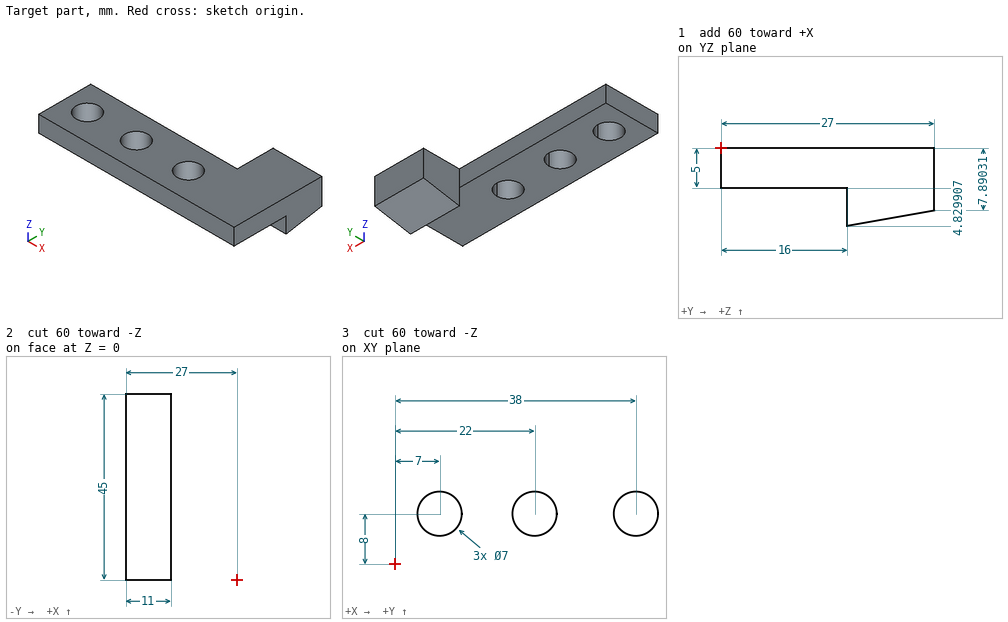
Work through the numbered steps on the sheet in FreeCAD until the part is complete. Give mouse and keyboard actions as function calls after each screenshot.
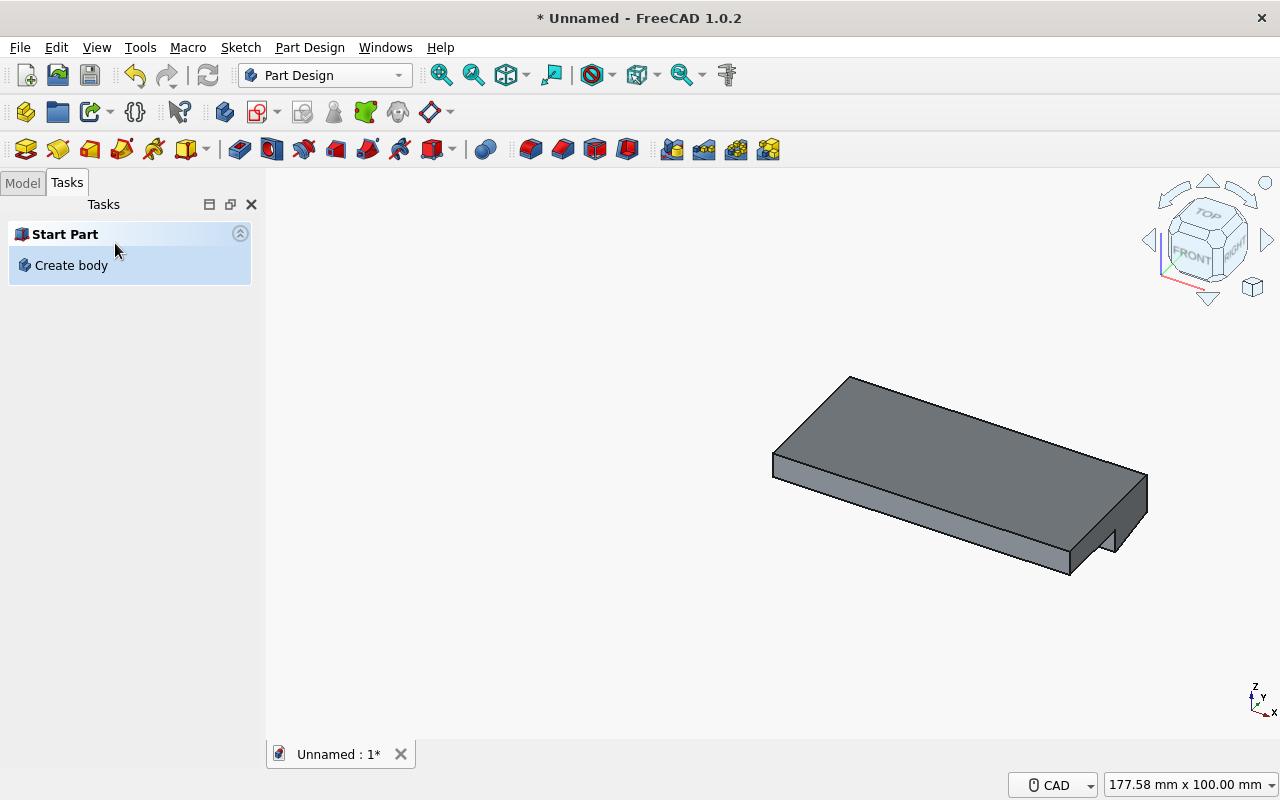
click(442, 76)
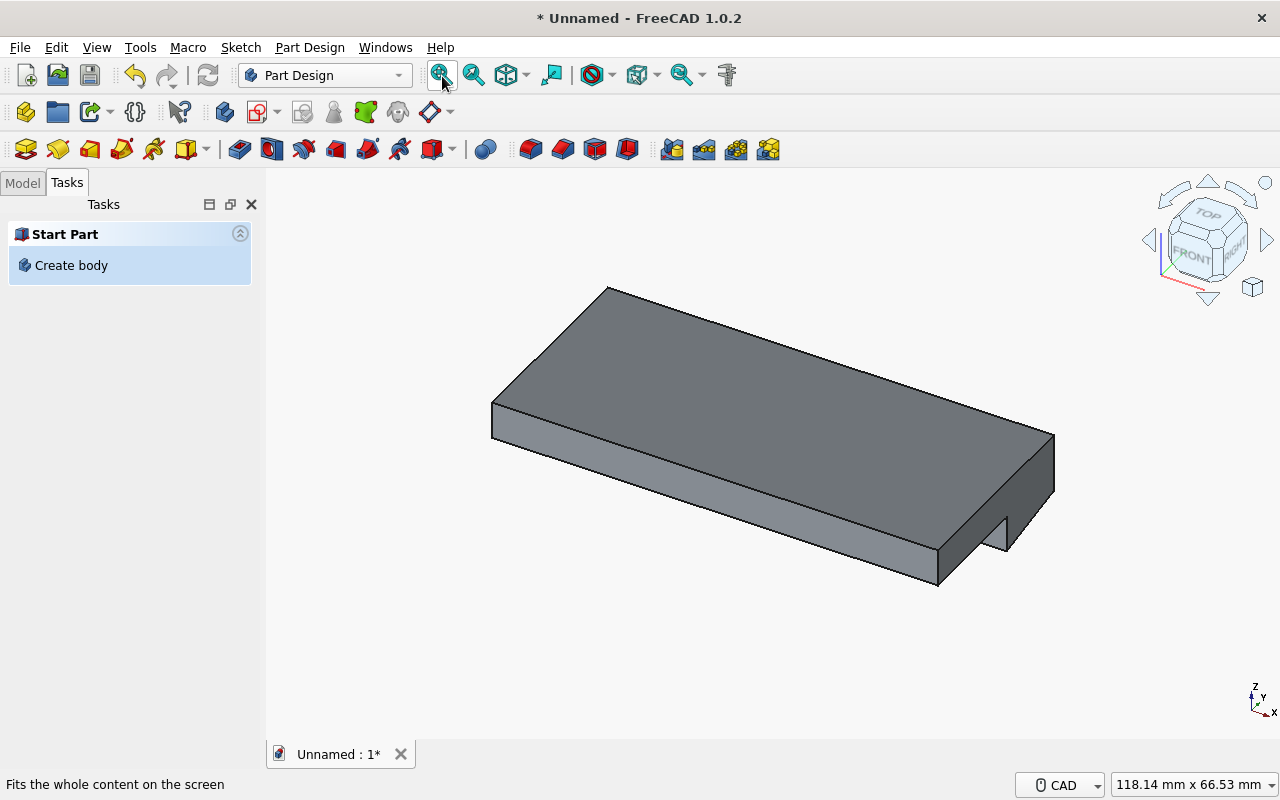
click(837, 439)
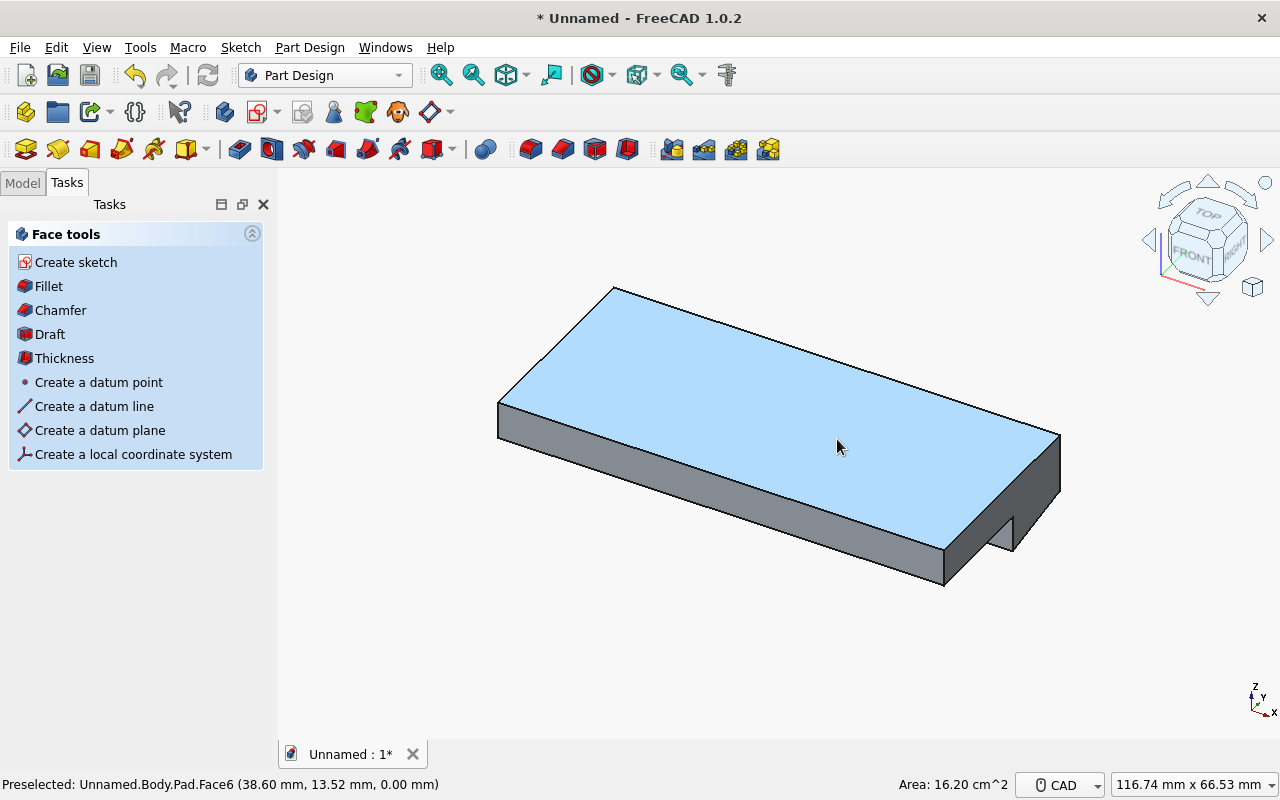
click(258, 112)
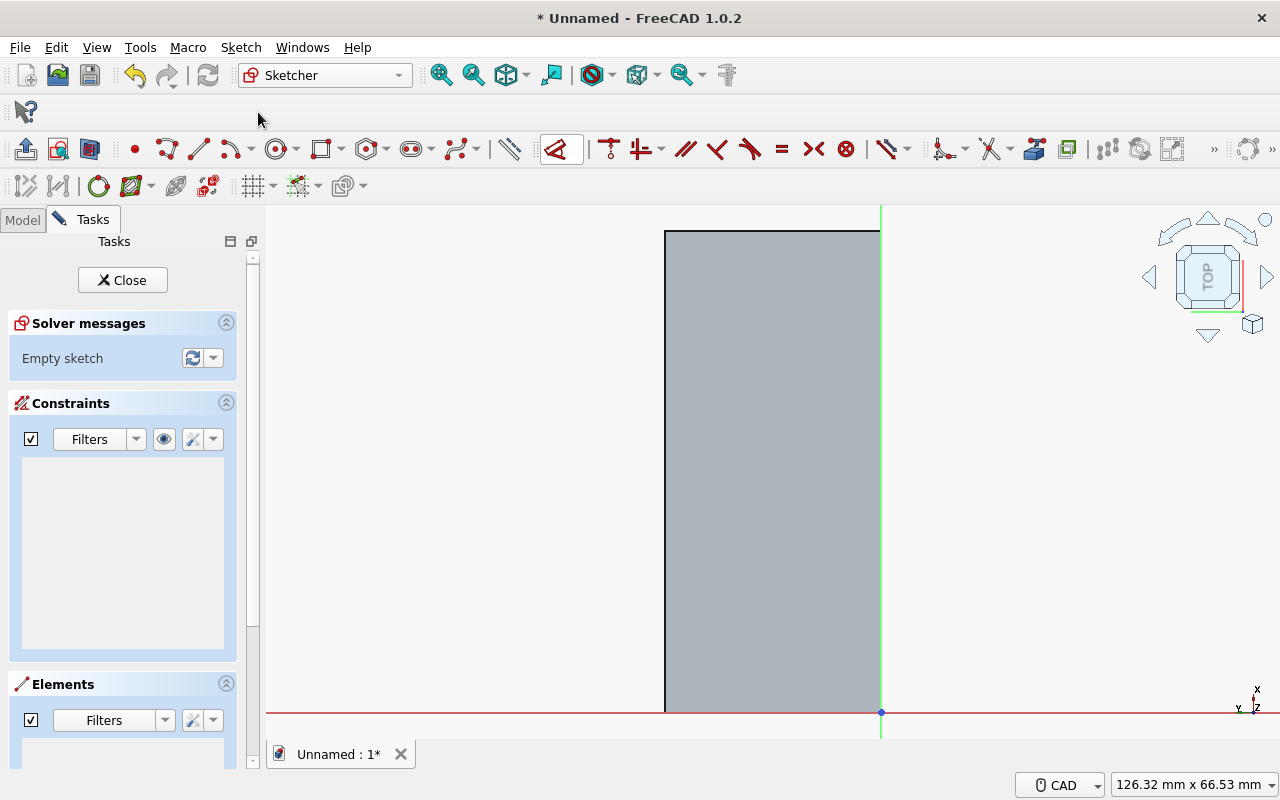
scroll(395, 233, down, 1)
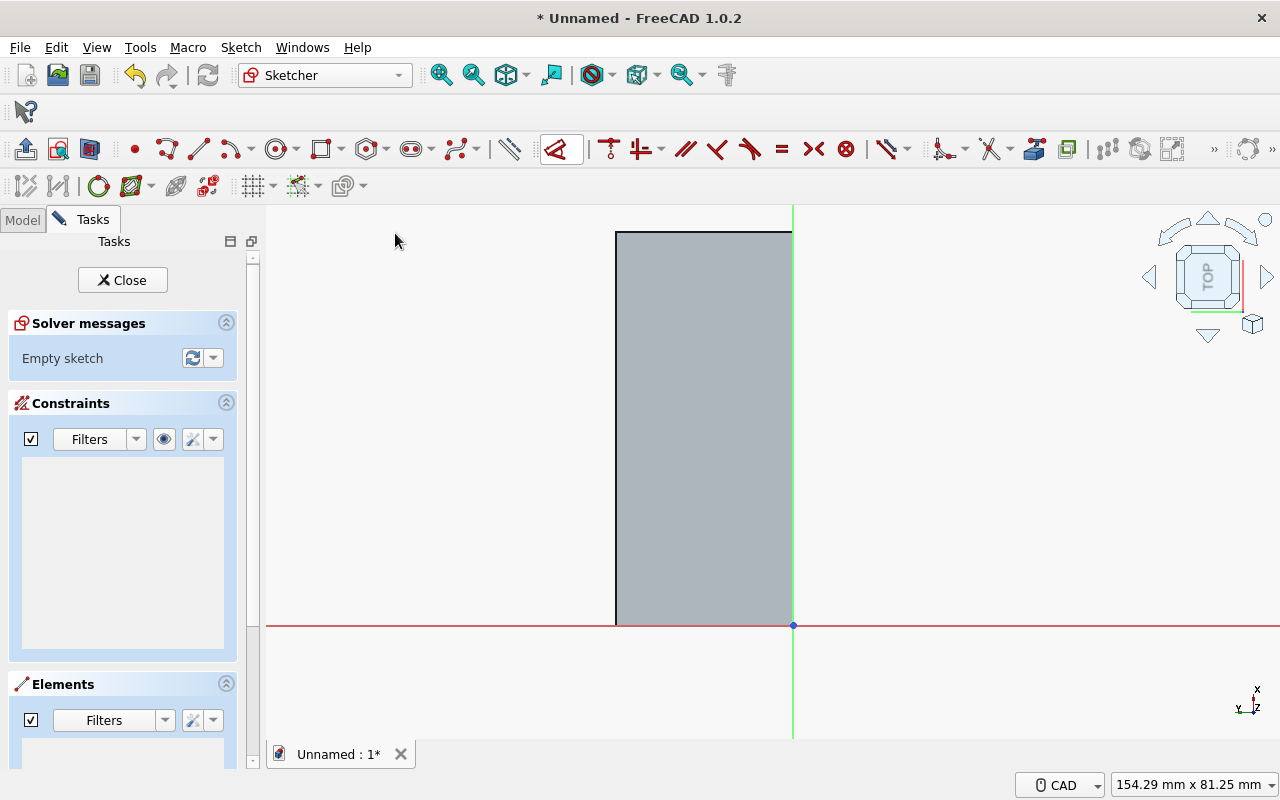
click(322, 150)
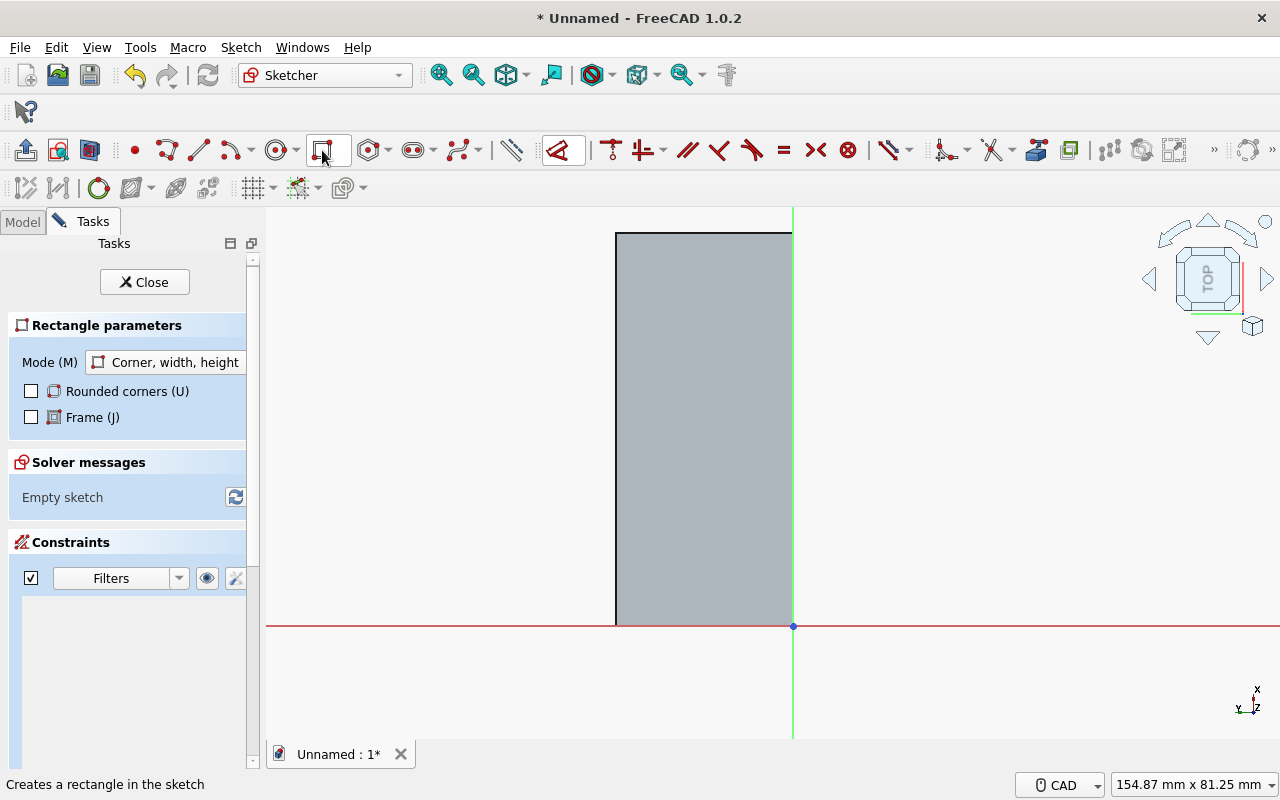
click(616, 332)
click(688, 626)
key(Escape)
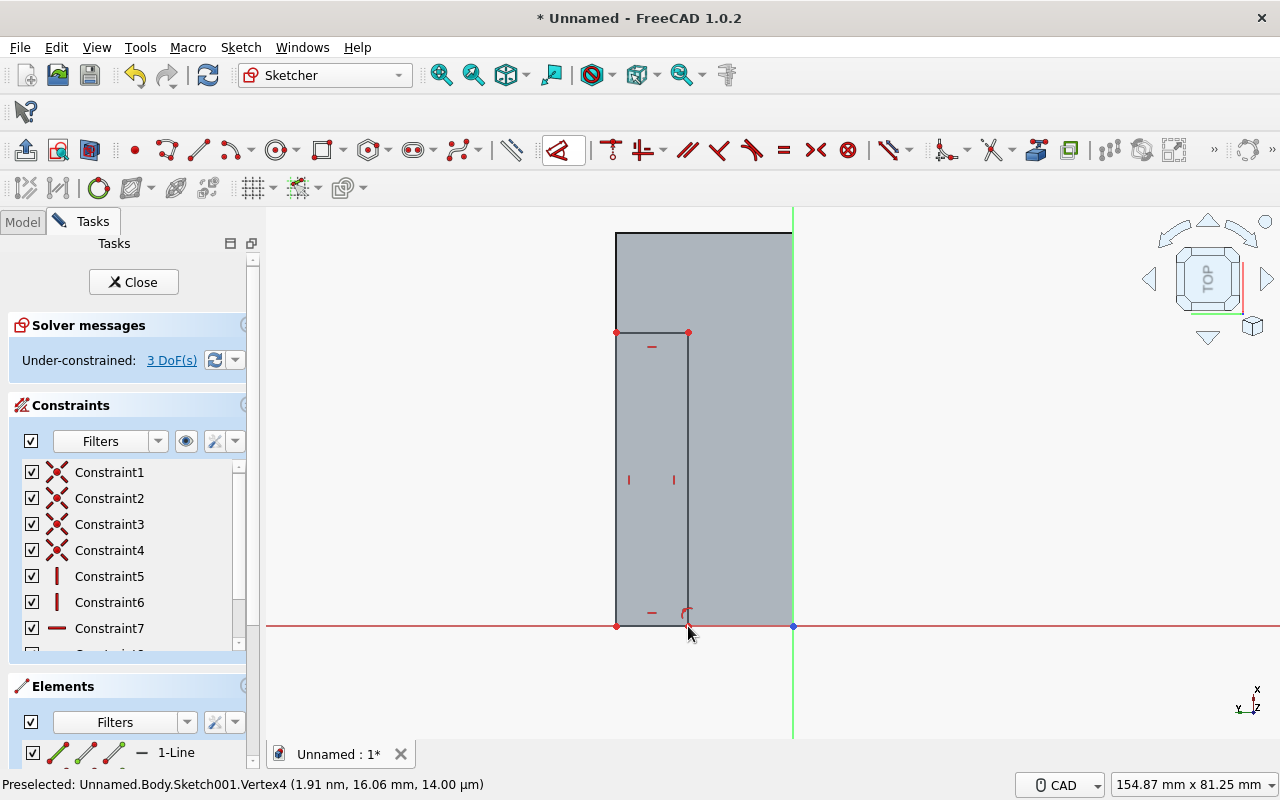
click(616, 421)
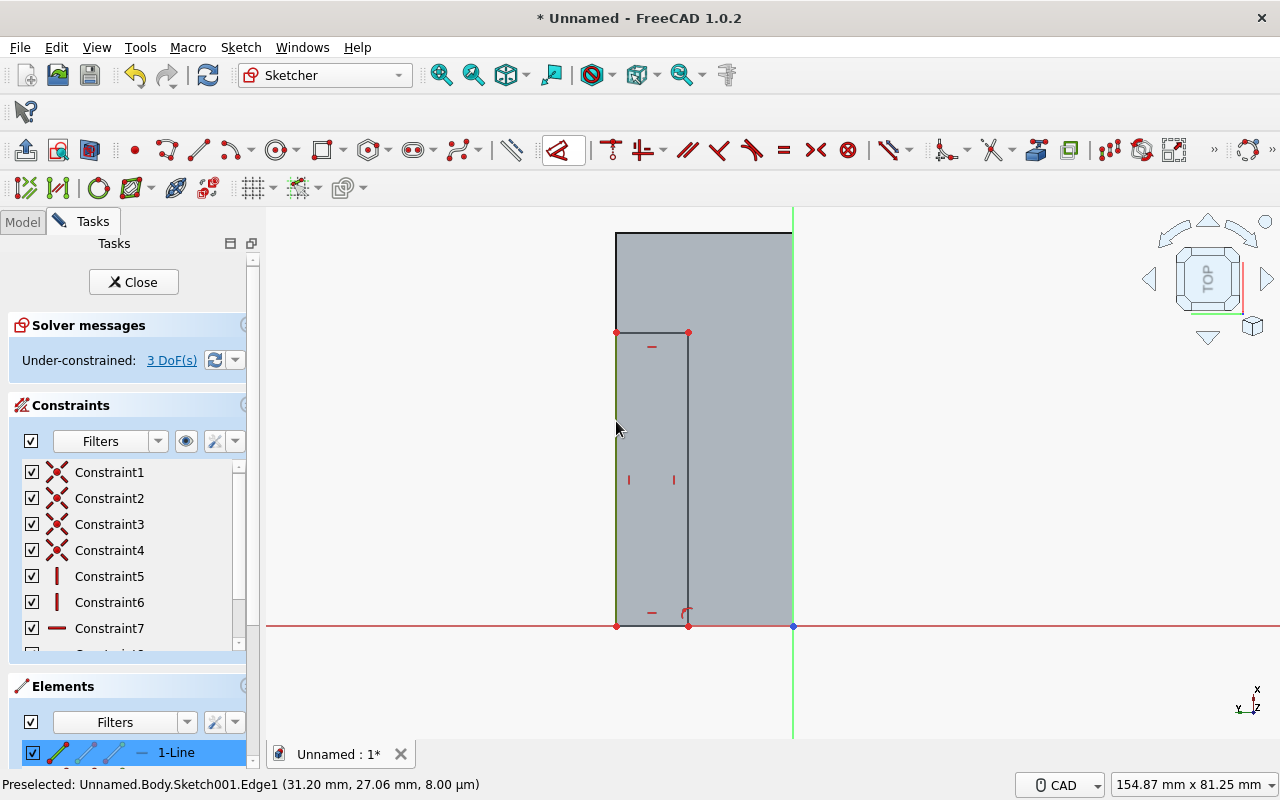
key(i)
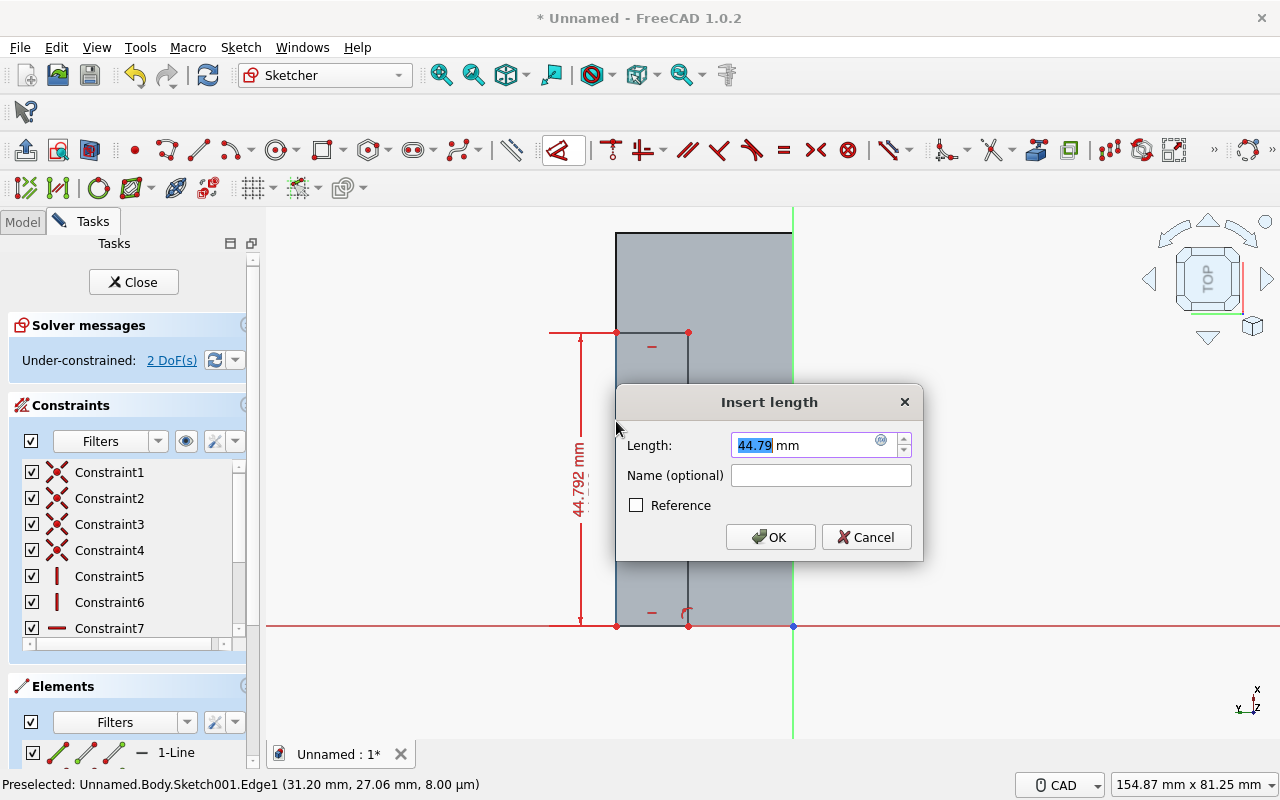
text(45)
key(Return)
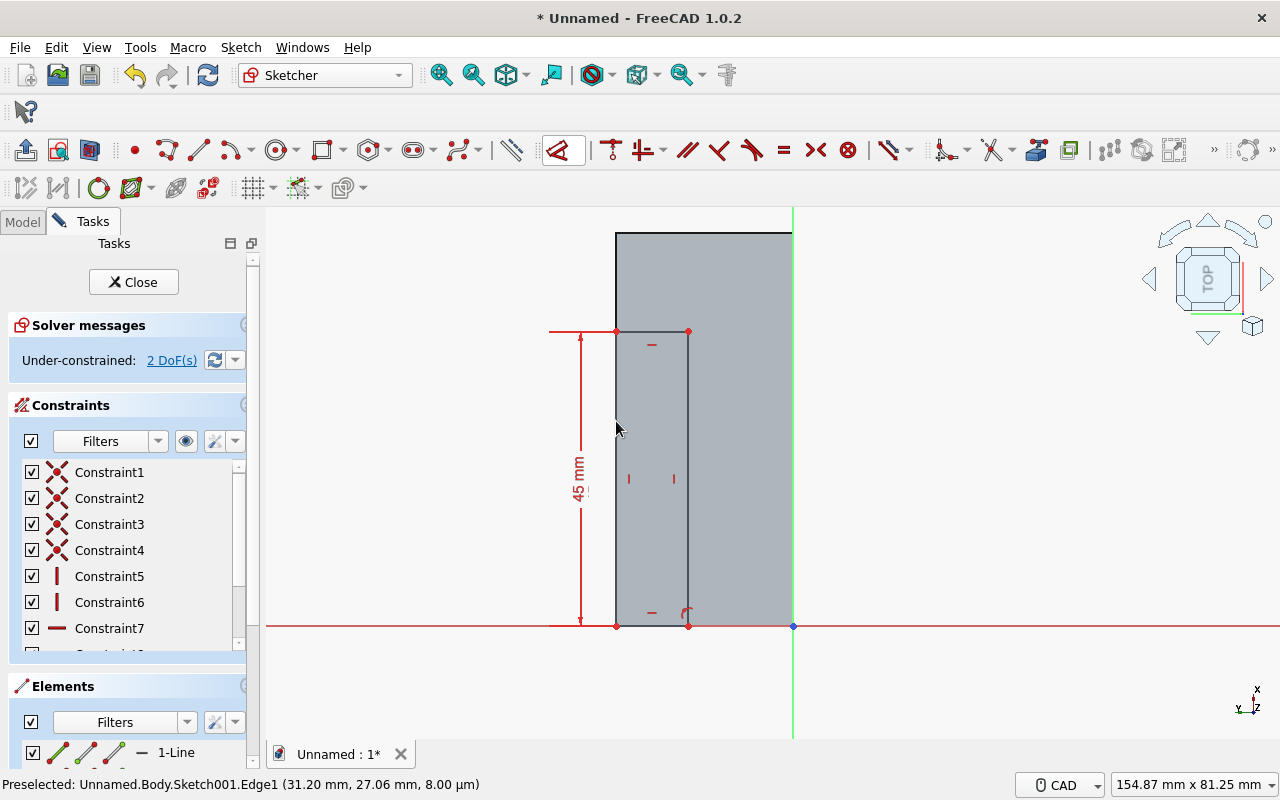
click(638, 626)